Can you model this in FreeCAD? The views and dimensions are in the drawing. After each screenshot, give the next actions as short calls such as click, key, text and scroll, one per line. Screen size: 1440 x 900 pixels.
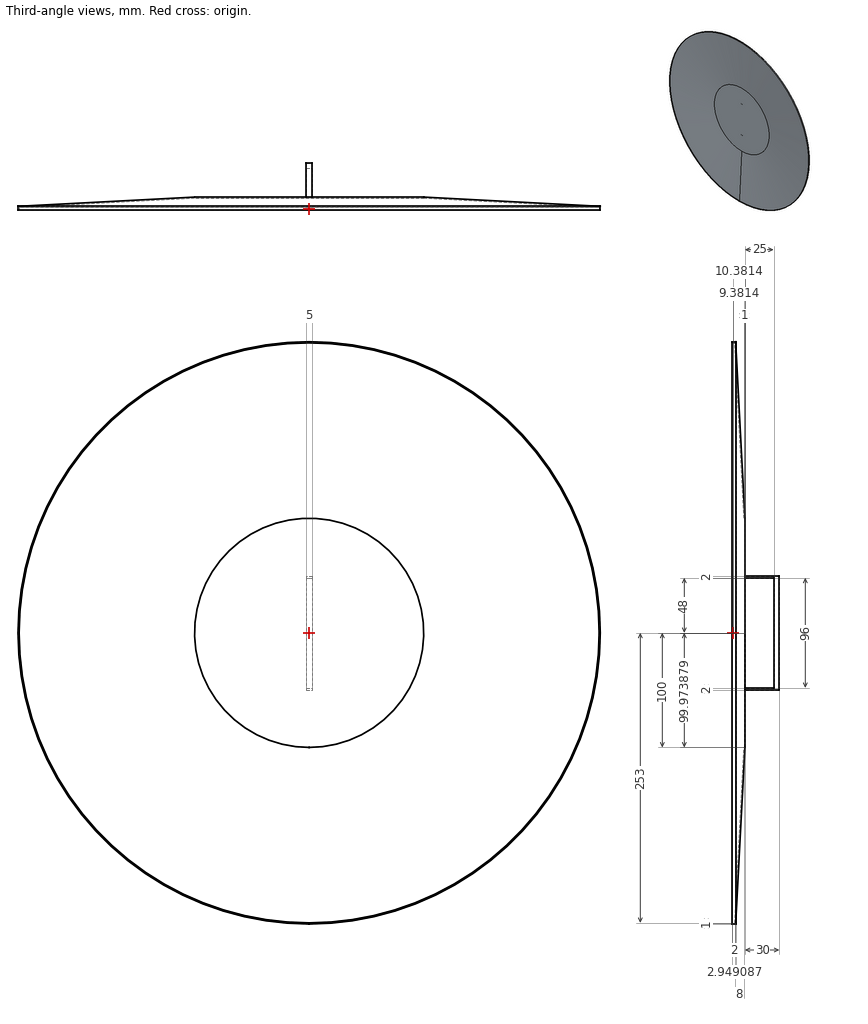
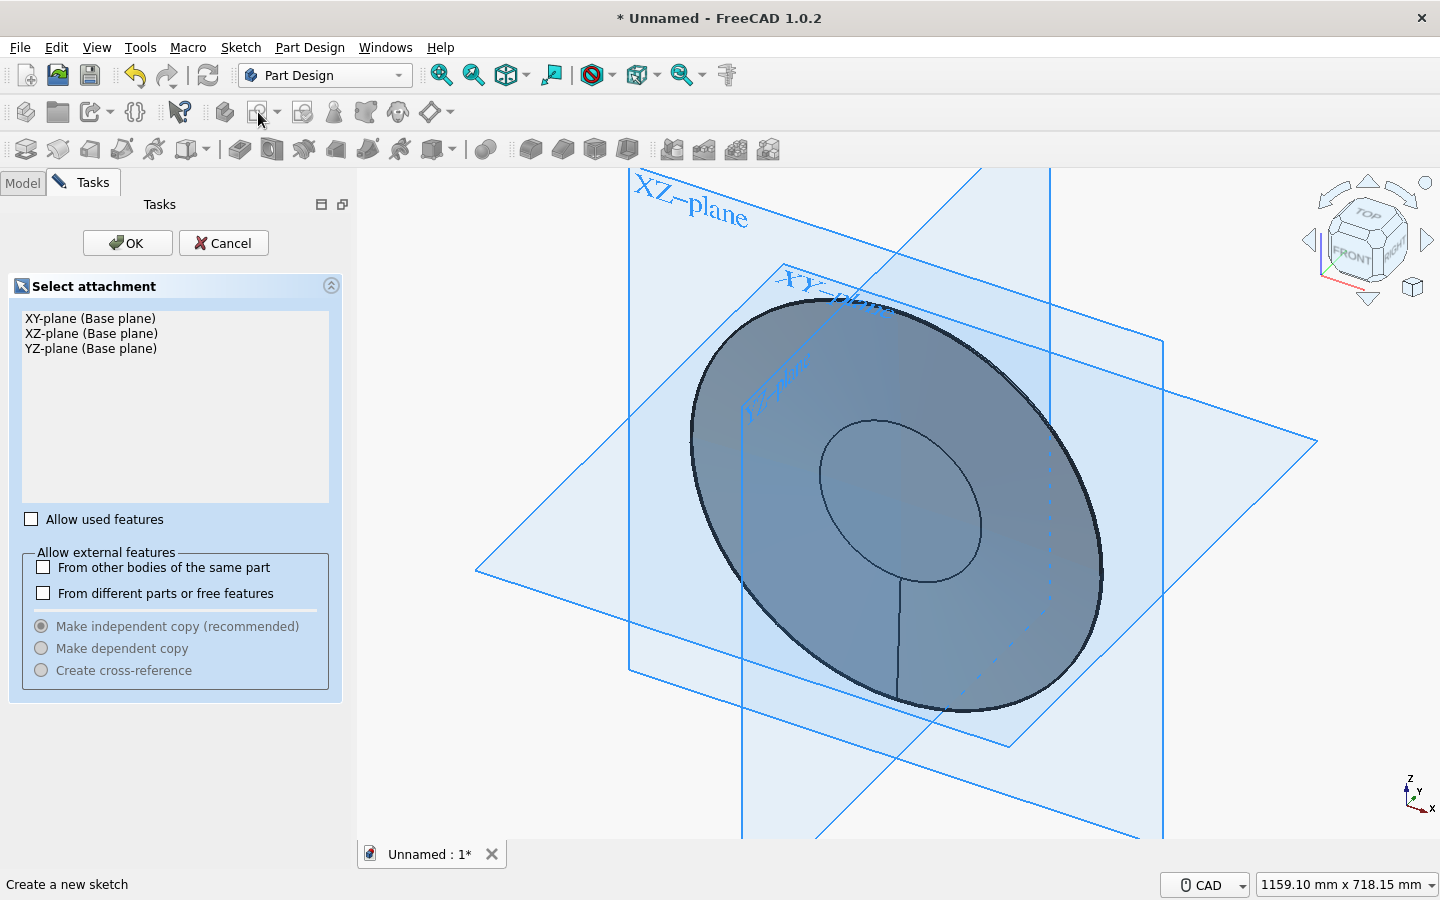
click(82, 348)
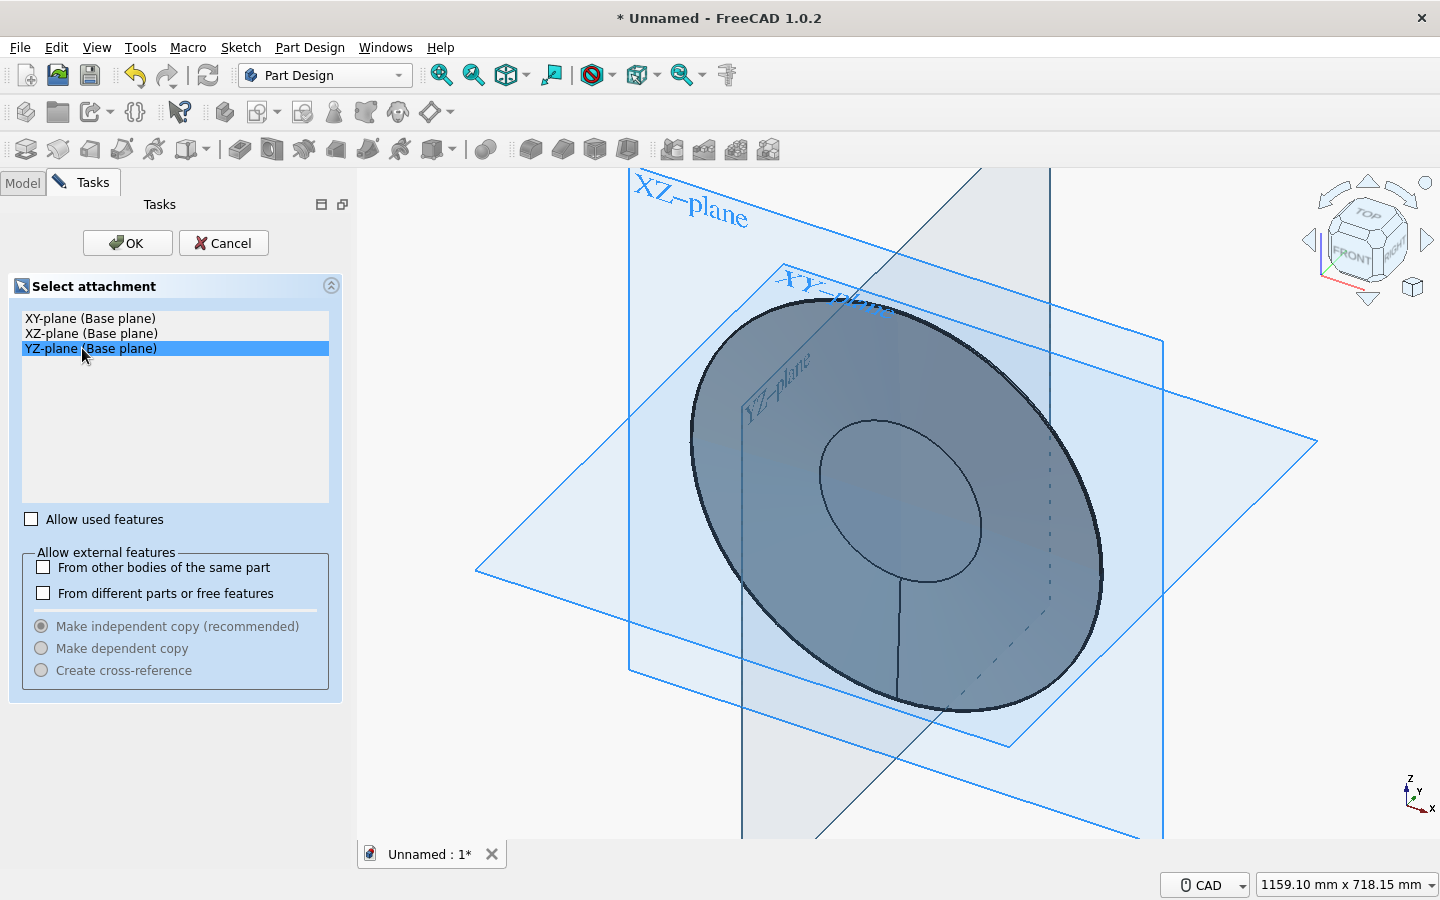
click(128, 243)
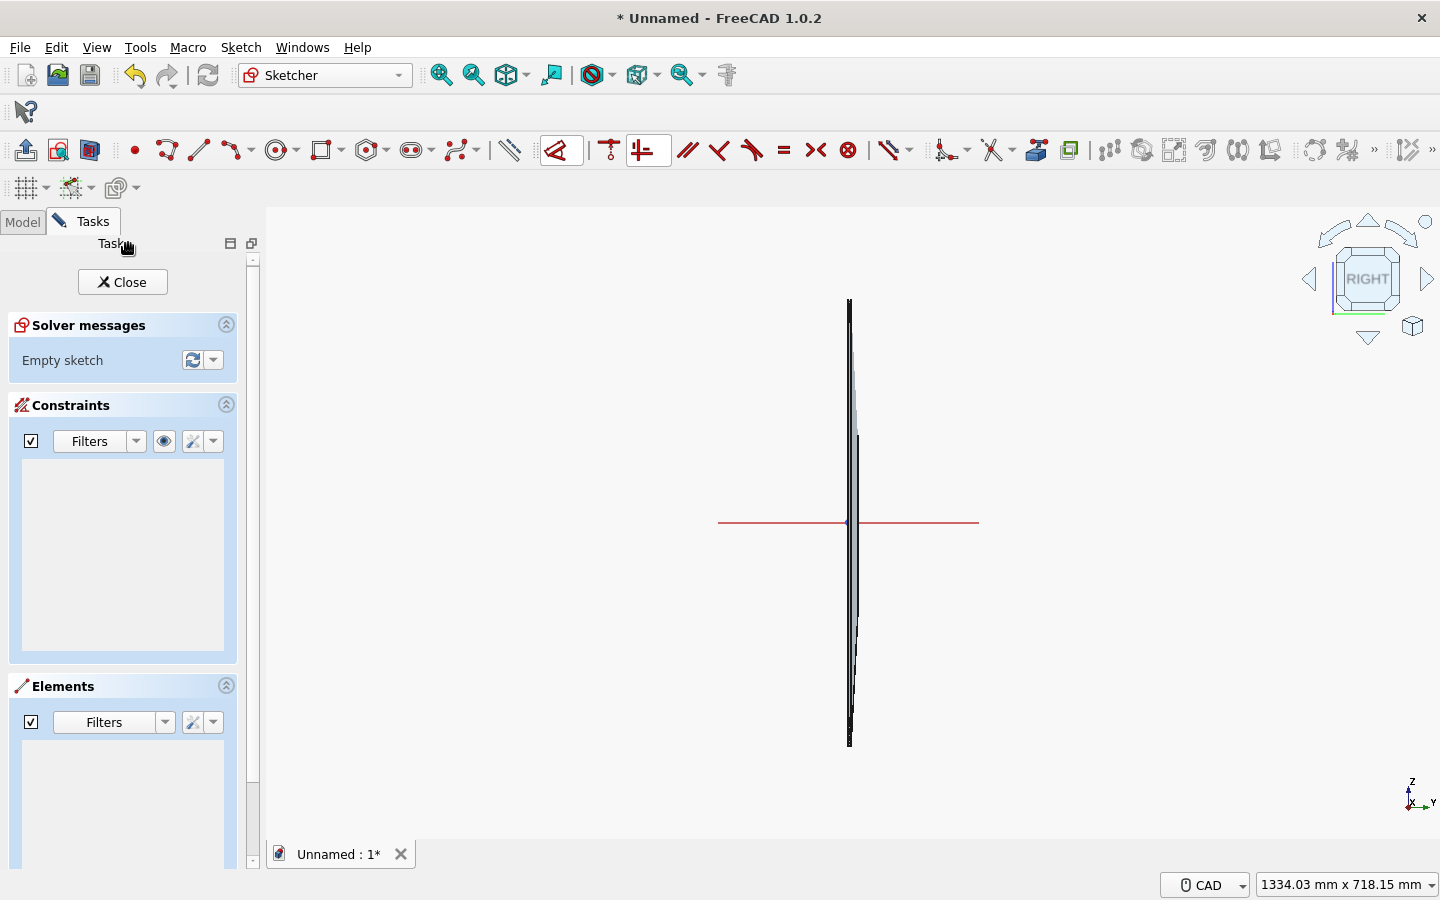
key(q)
key(s)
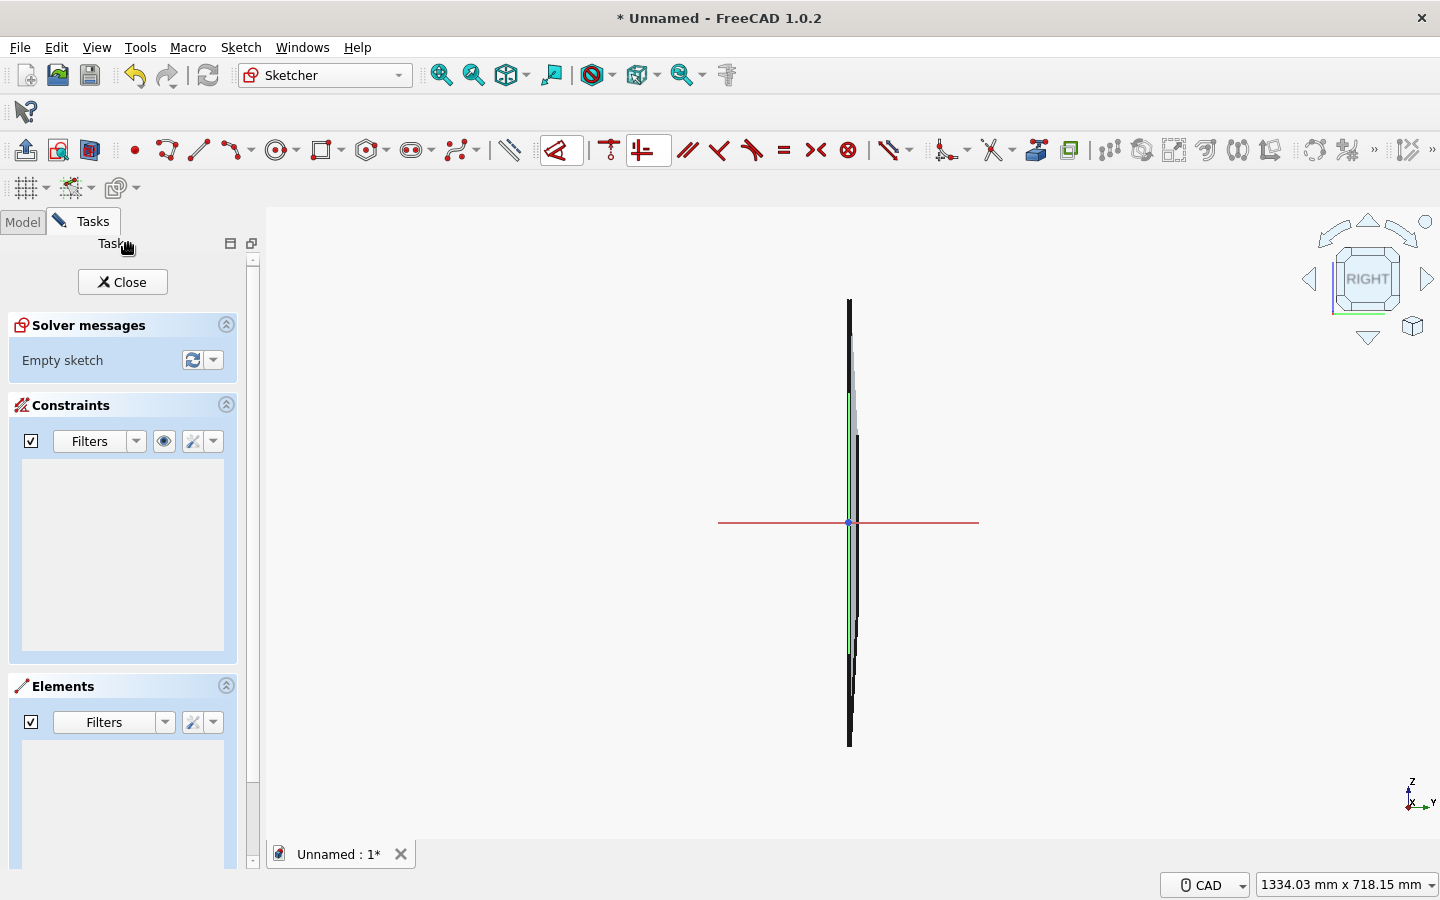
scroll(887, 523, up, 8)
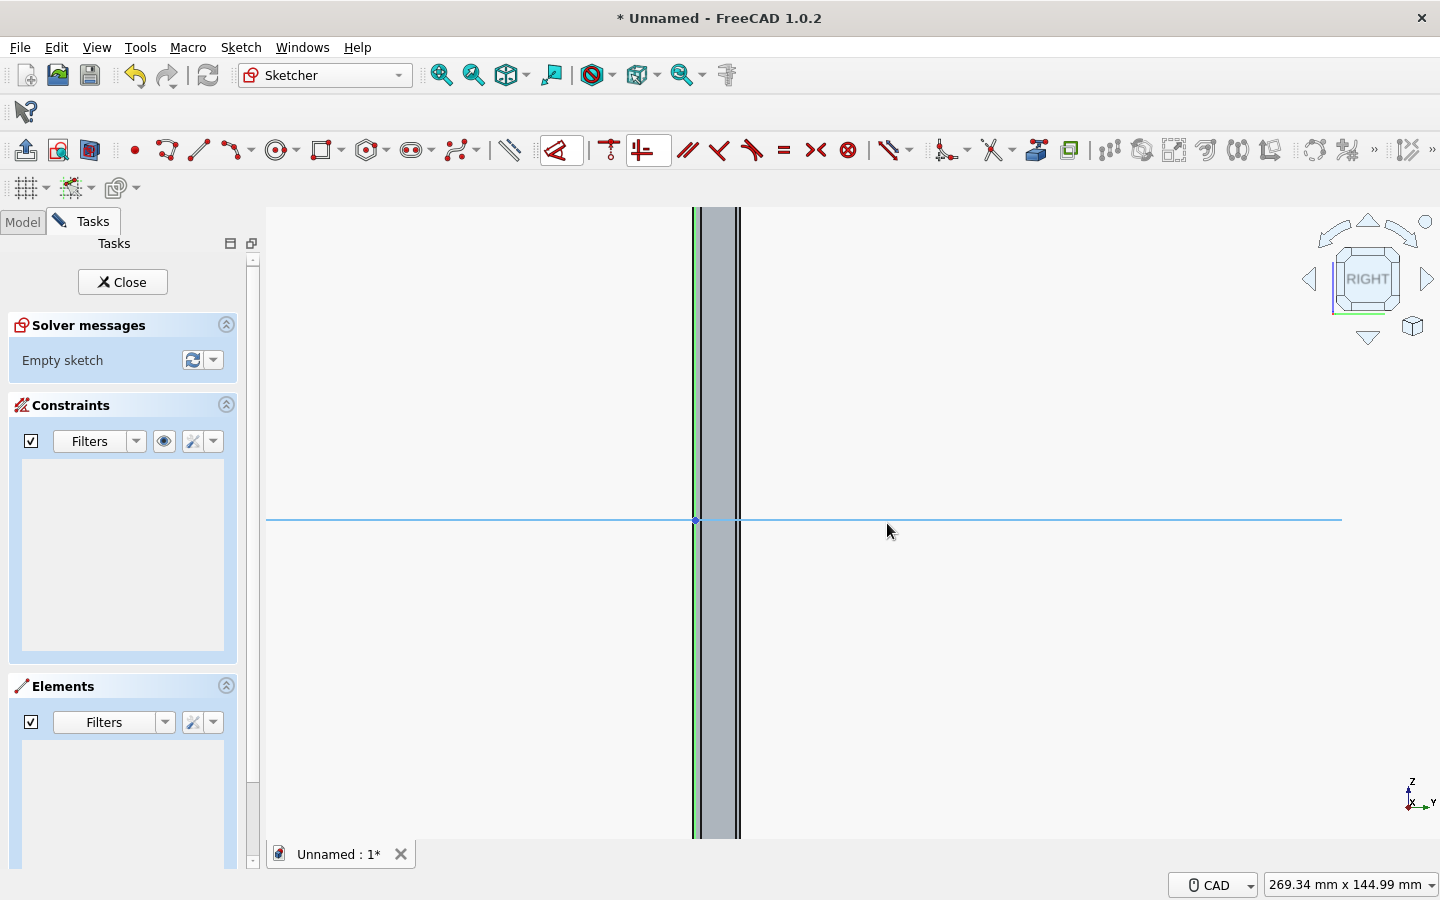
click(168, 150)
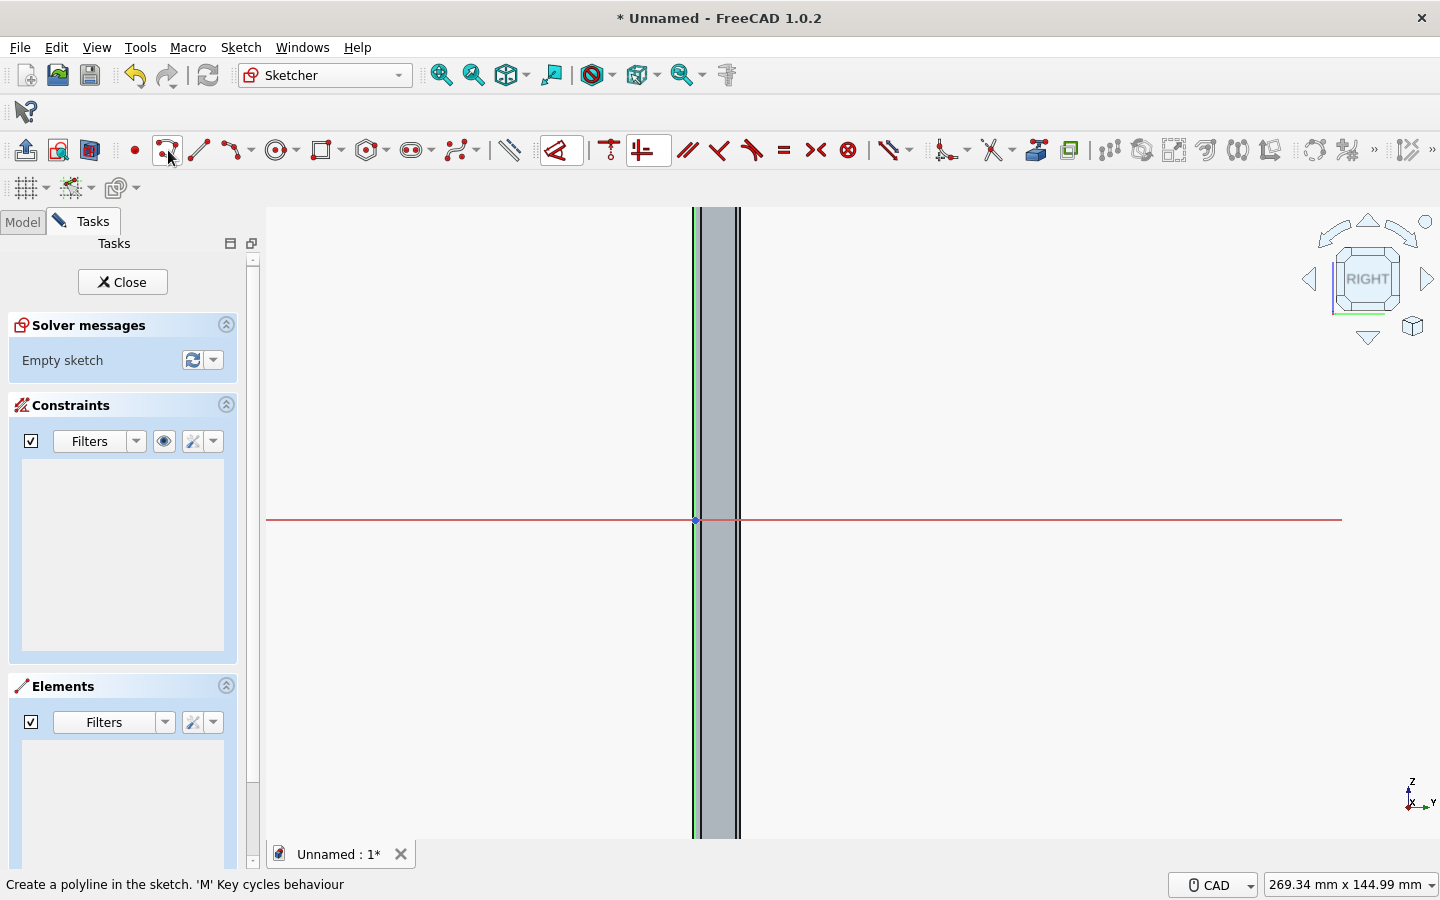
click(740, 311)
click(849, 311)
click(849, 730)
click(740, 730)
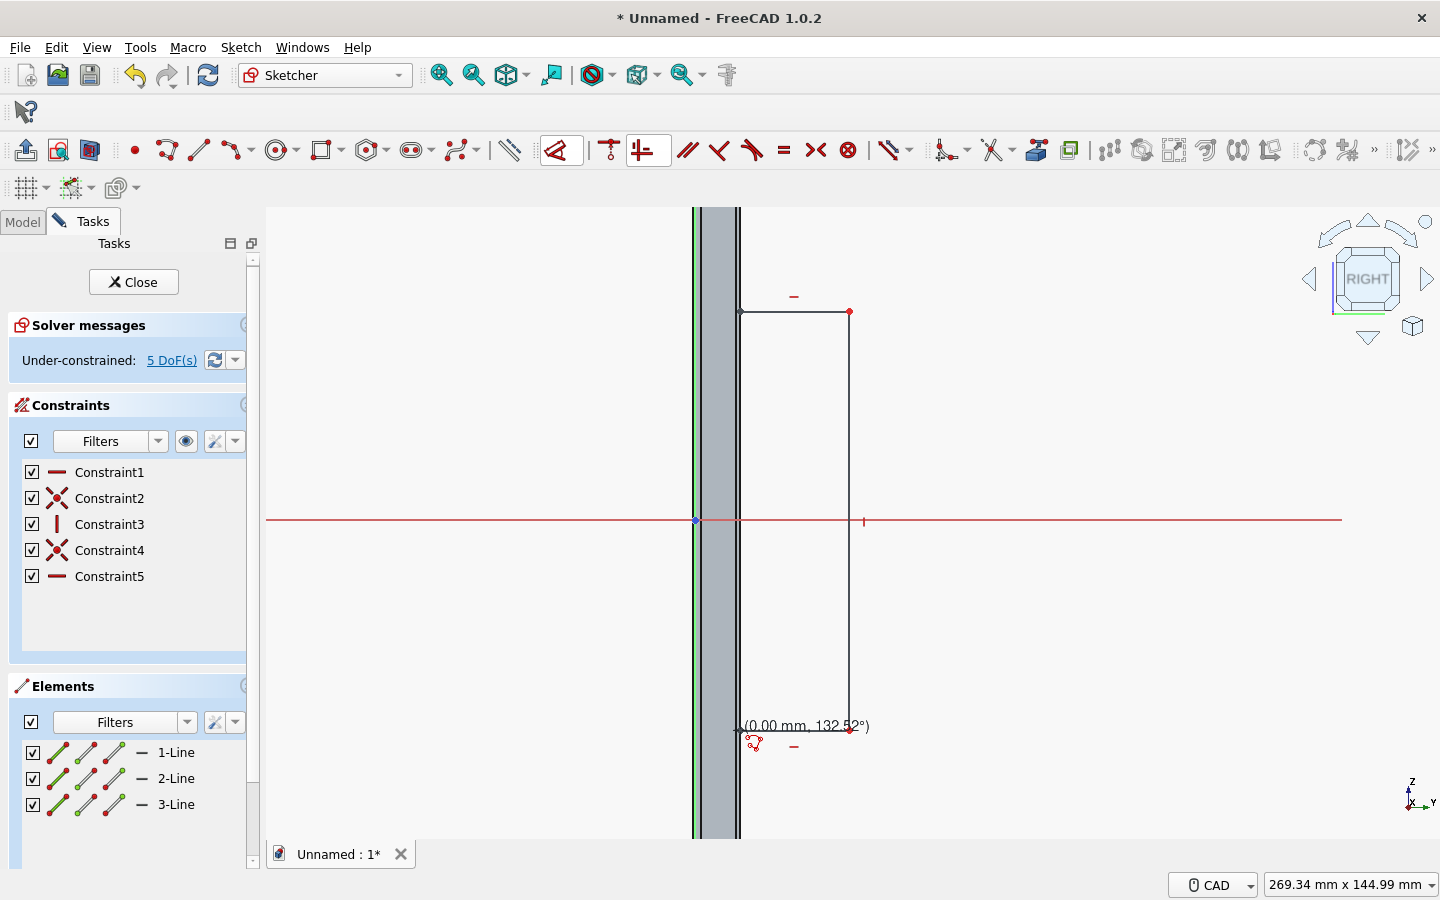
scroll(740, 738, up, 3)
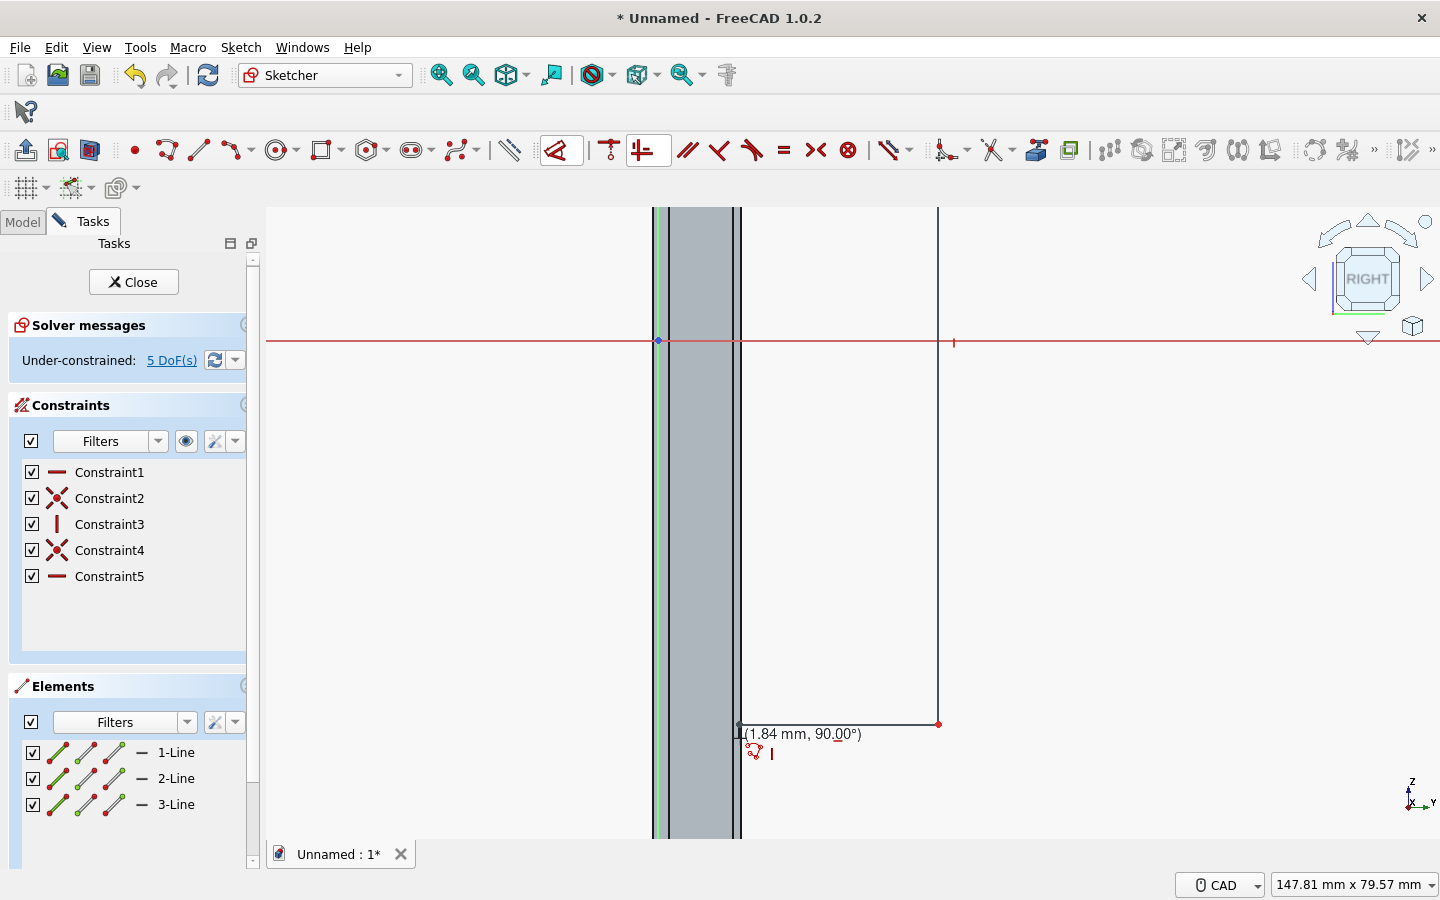
click(740, 738)
click(979, 738)